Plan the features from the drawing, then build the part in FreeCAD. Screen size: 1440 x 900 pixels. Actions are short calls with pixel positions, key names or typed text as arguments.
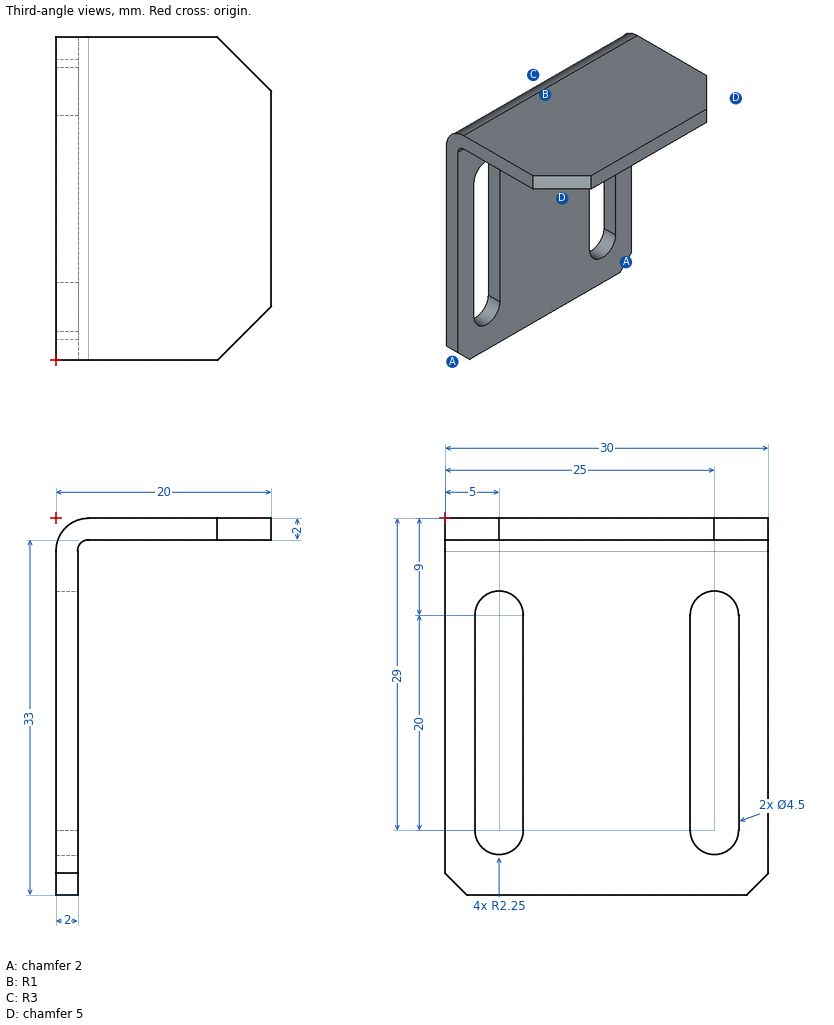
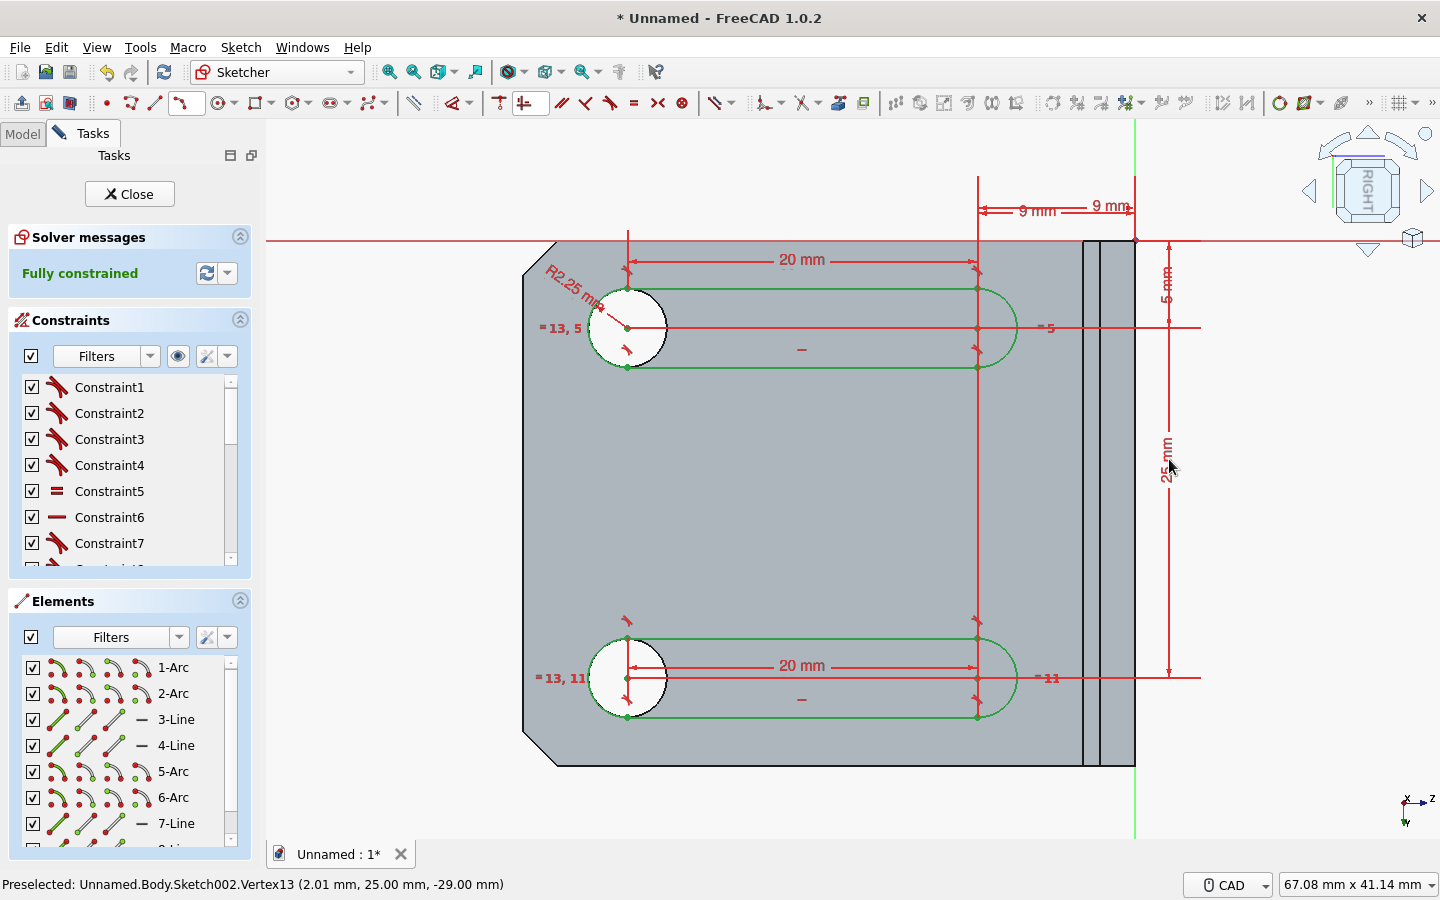
click(130, 194)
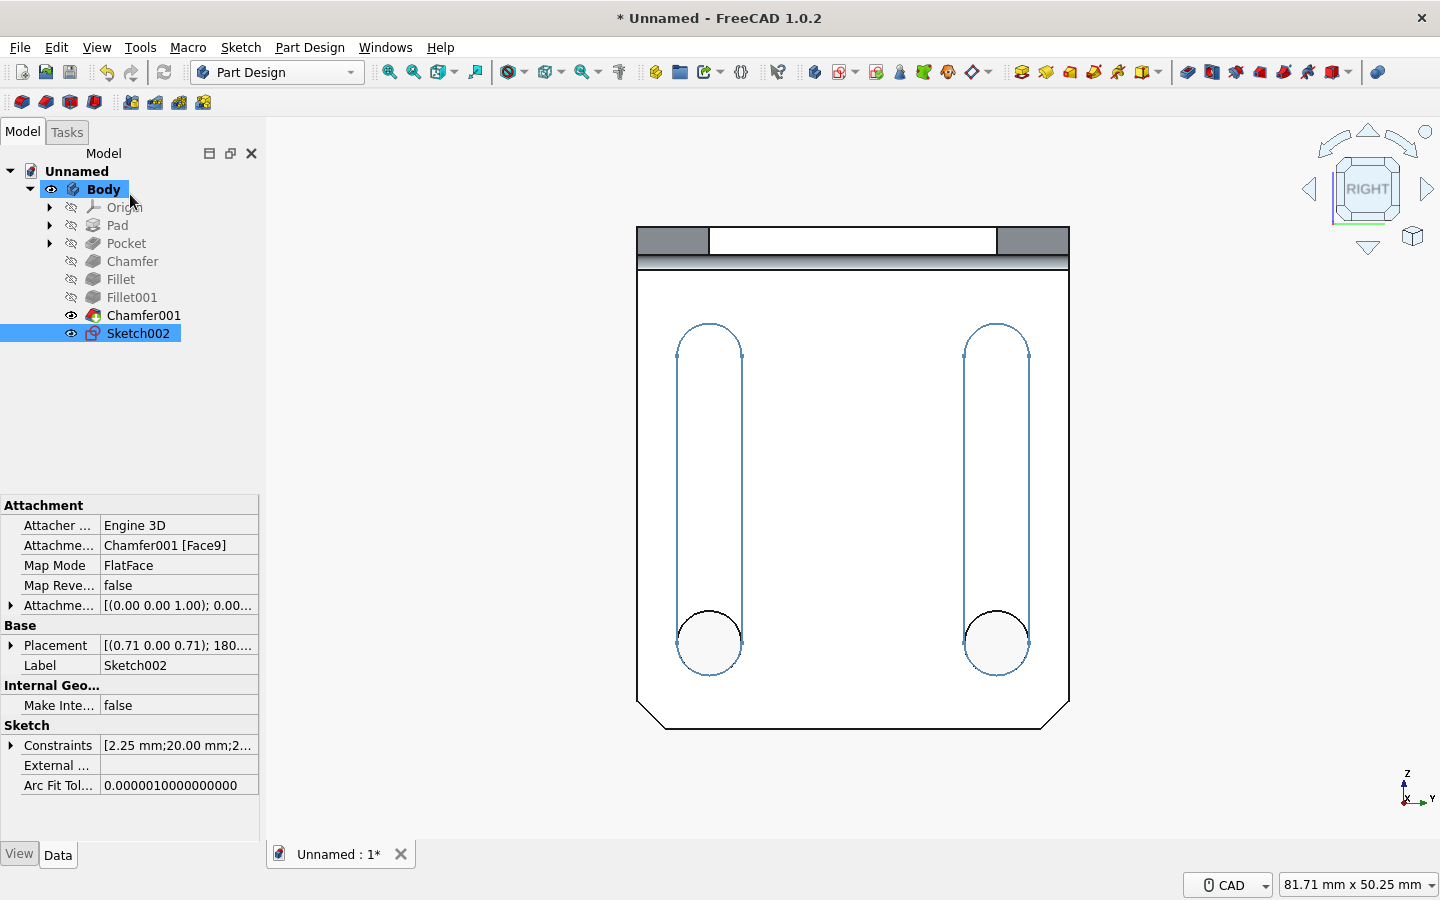
click(1188, 72)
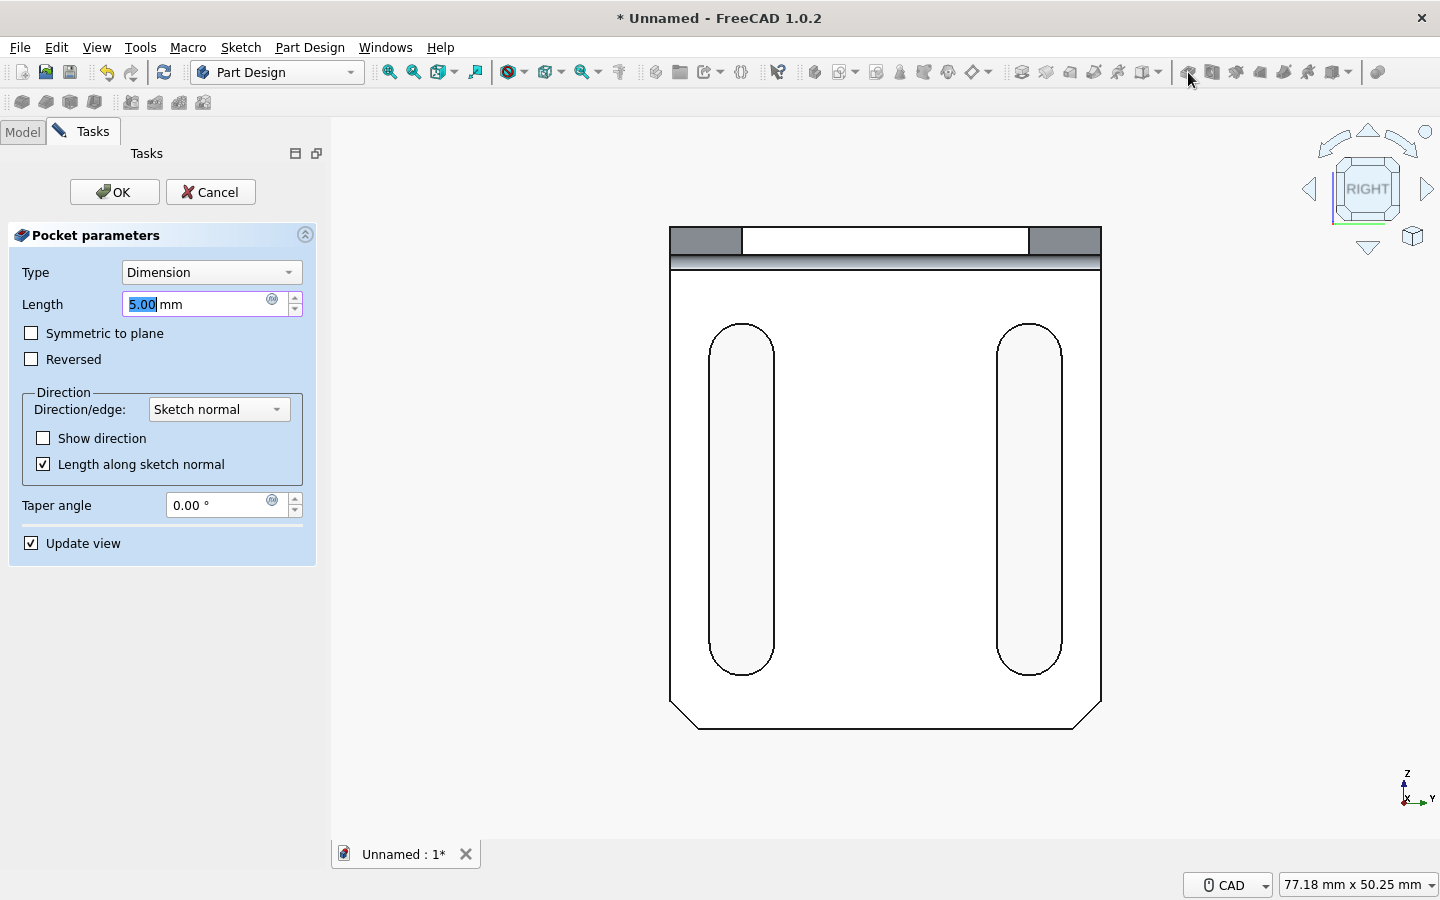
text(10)
key(Tab)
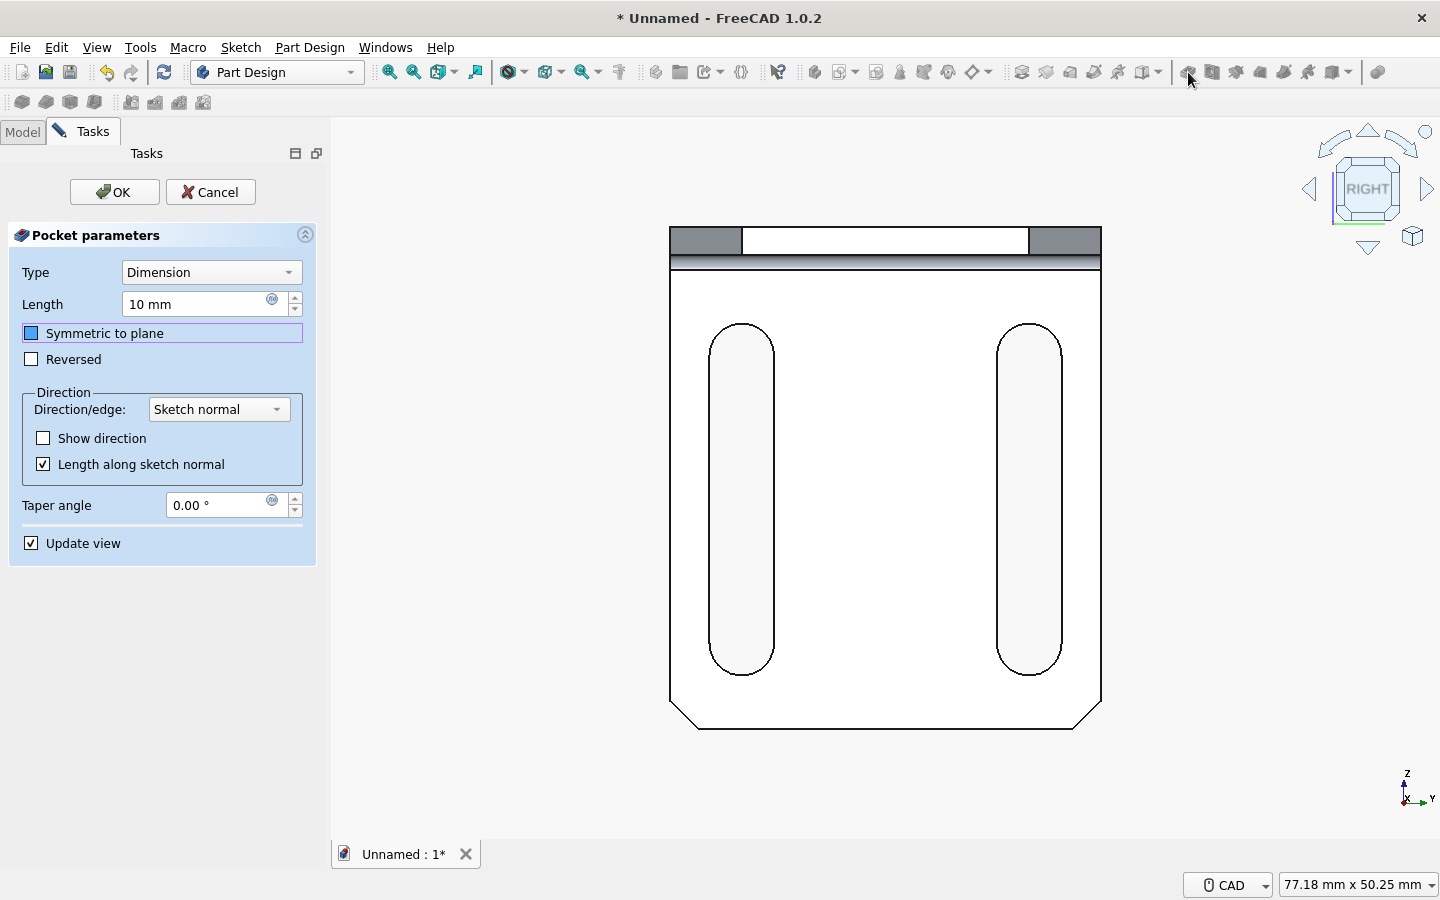
click(115, 192)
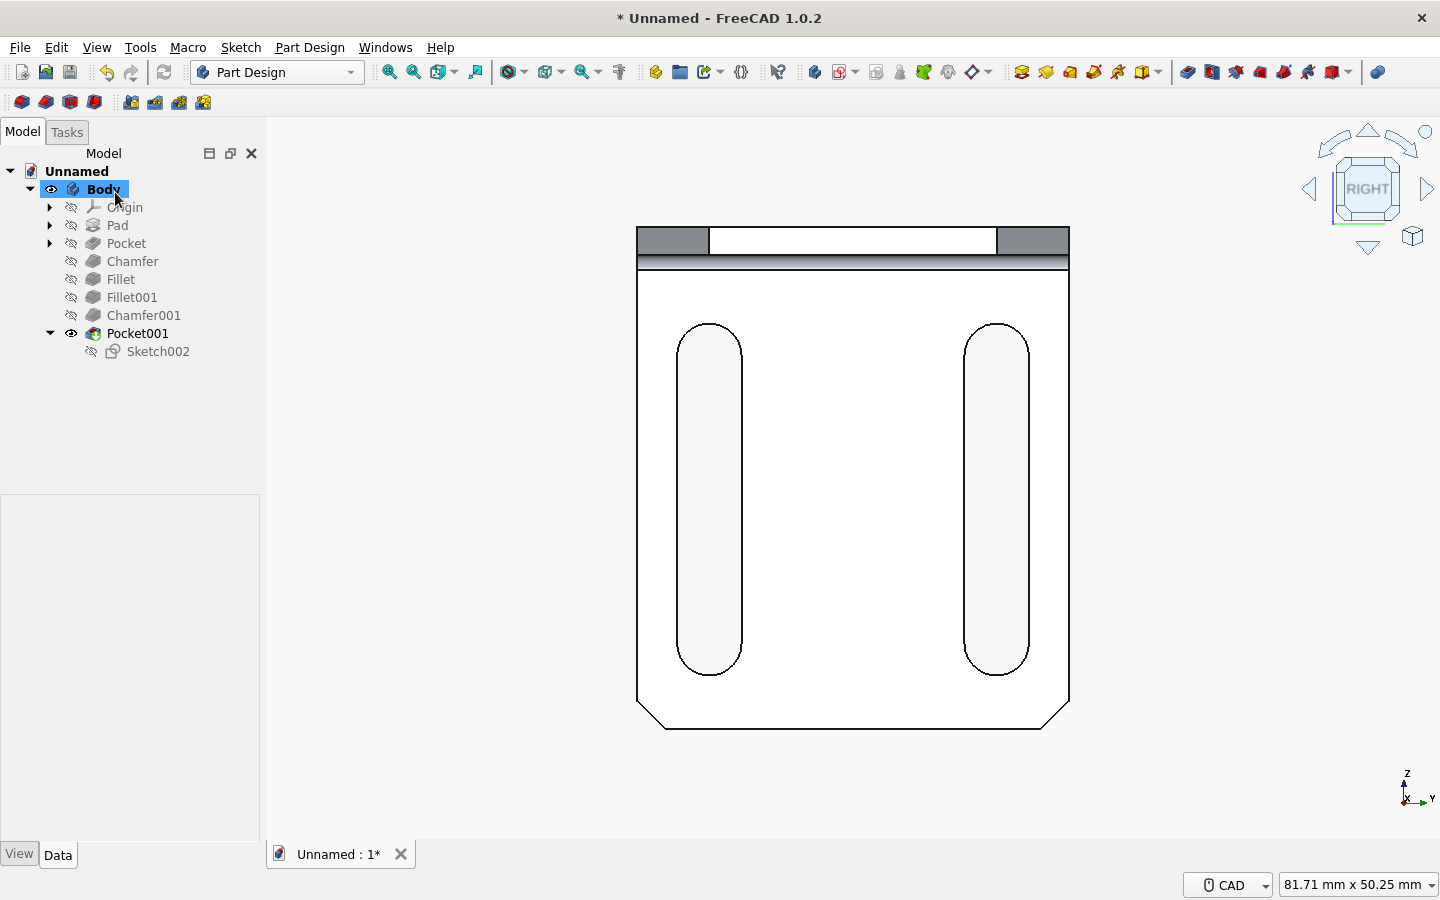
key(0)